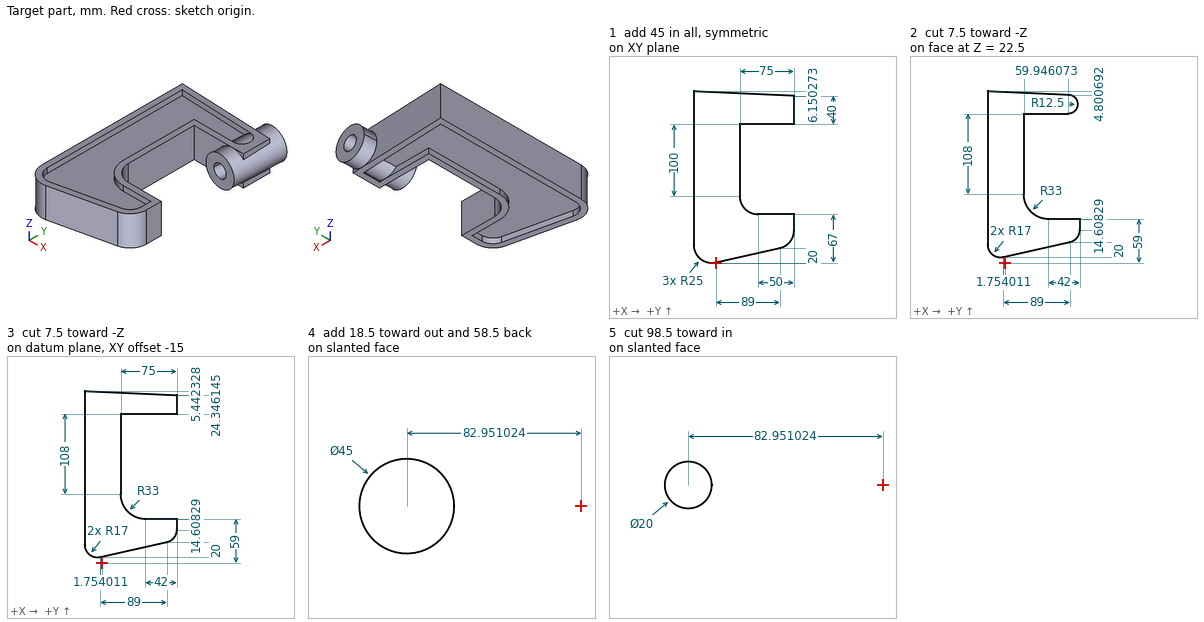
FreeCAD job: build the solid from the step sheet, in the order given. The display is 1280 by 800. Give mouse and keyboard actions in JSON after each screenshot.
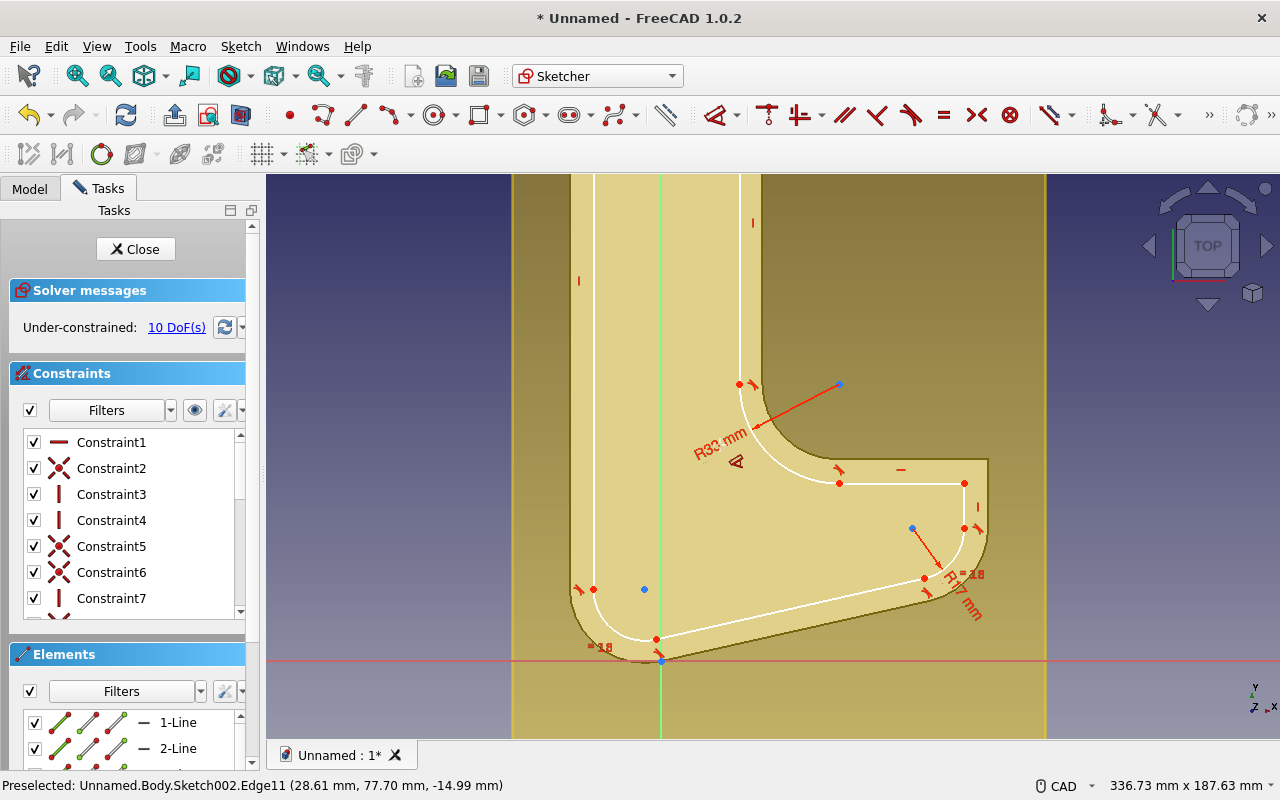
{"action": "left_click", "coordinate": [877, 484]}
{"action": "left_click", "coordinate": [902, 518]}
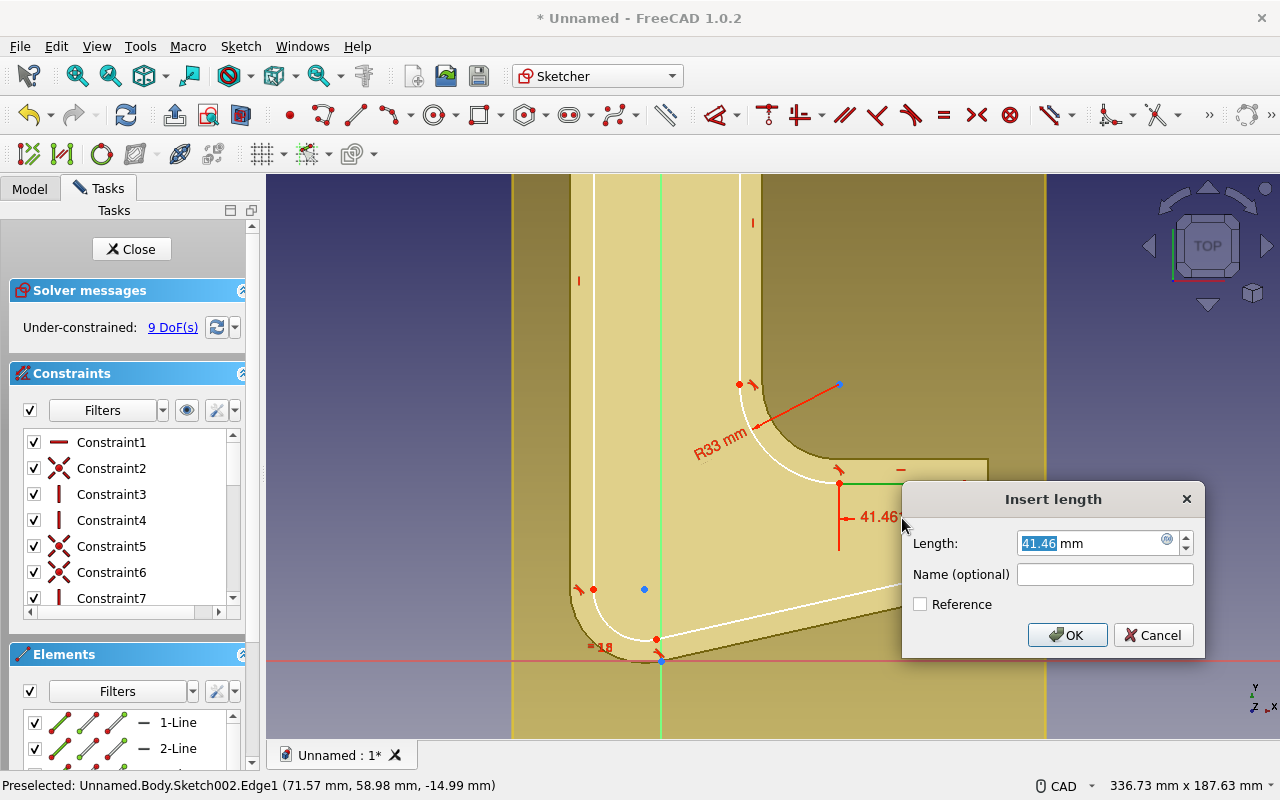
{"action": "type", "text": "42"}
{"action": "key", "text": "Return"}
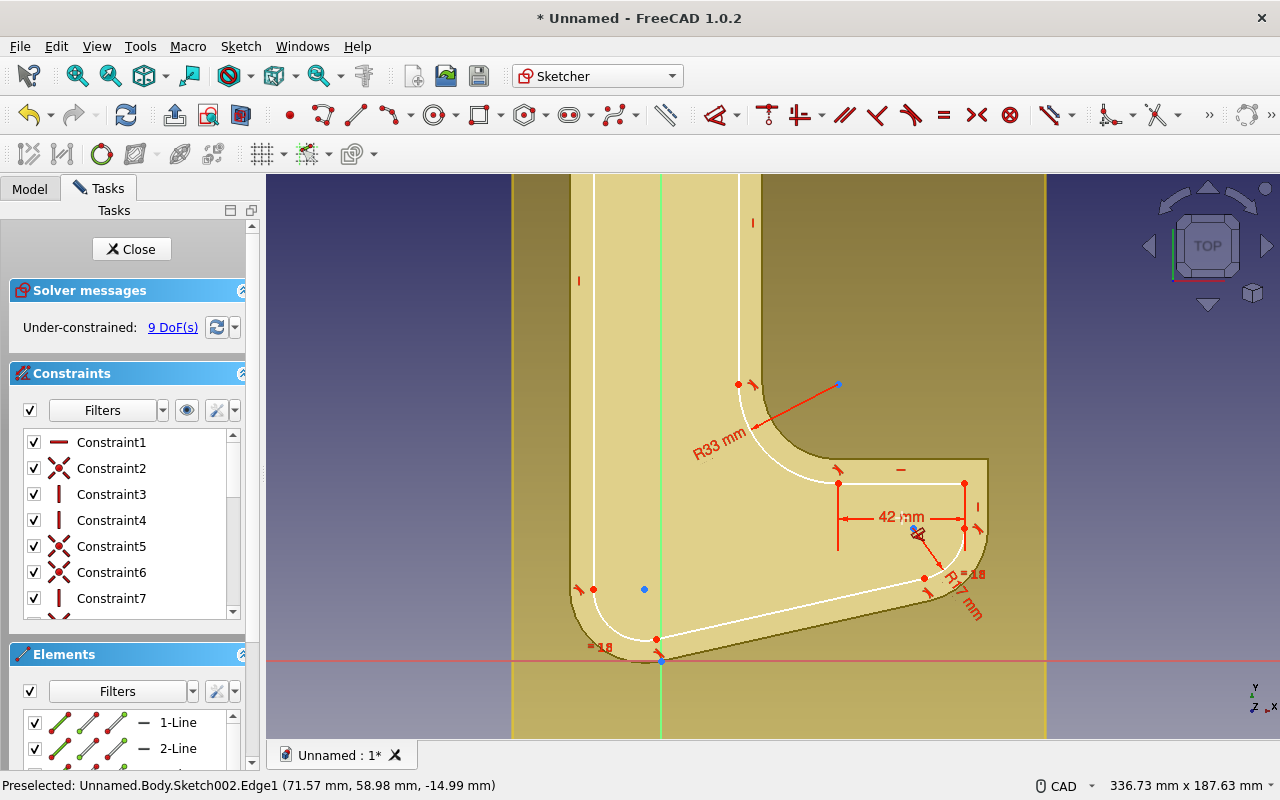
{"action": "scroll", "coordinate": [614, 628], "scroll_direction": "down", "scroll_amount": 3}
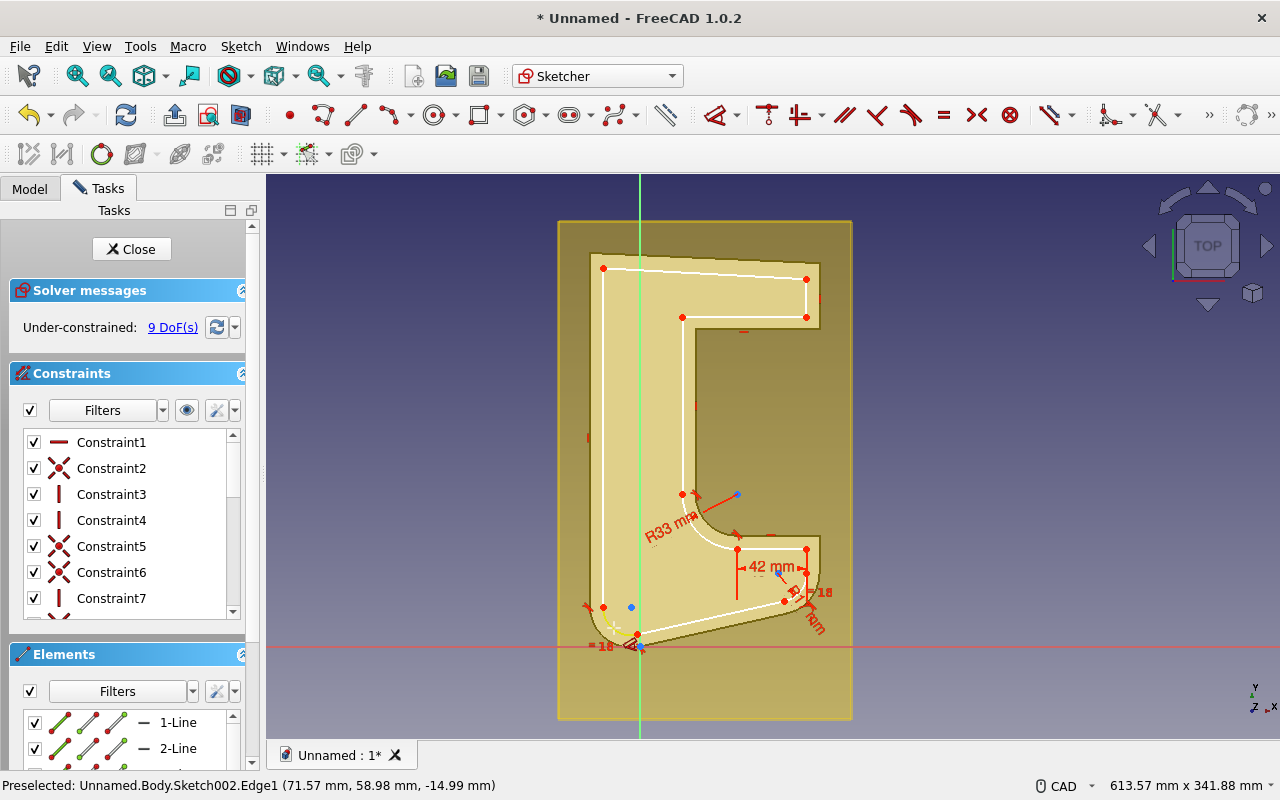
{"action": "left_click", "coordinate": [769, 317]}
{"action": "left_click", "coordinate": [744, 351]}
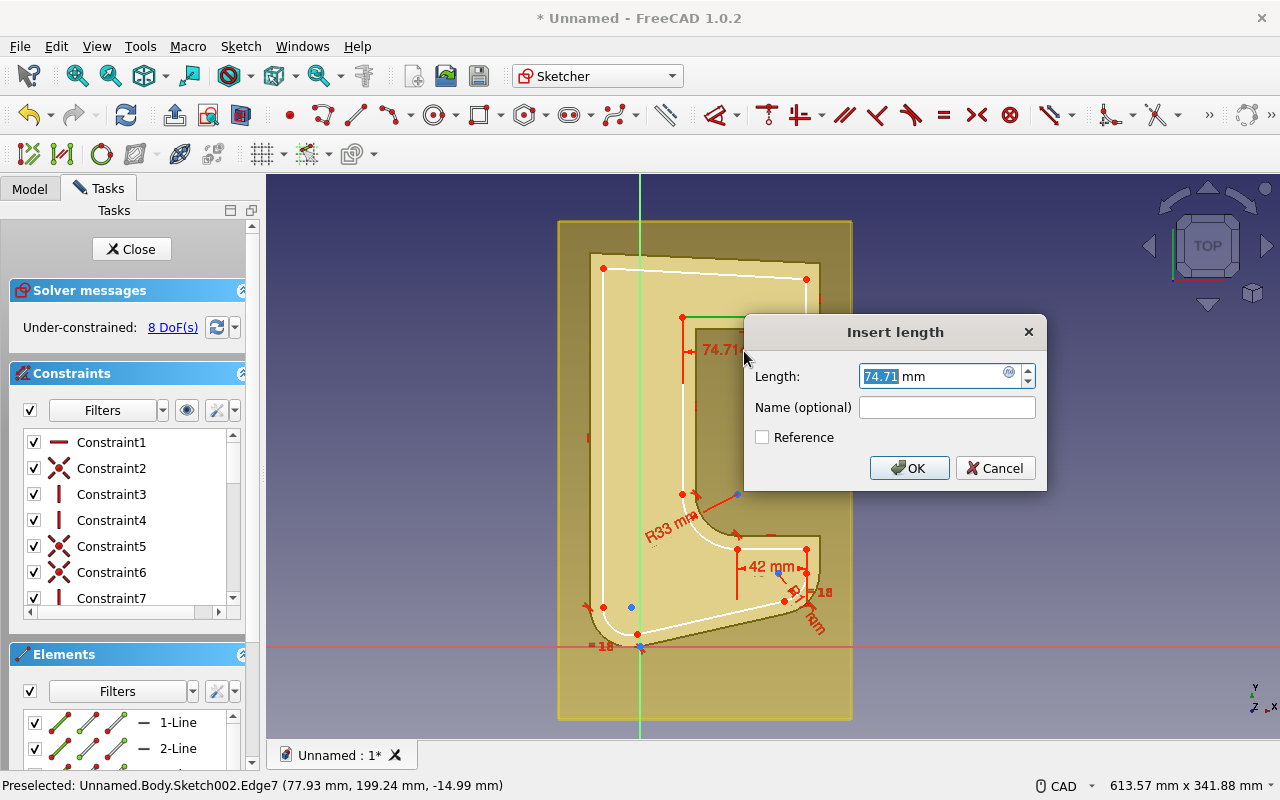
{"action": "type", "text": "75"}
{"action": "key", "text": "Return"}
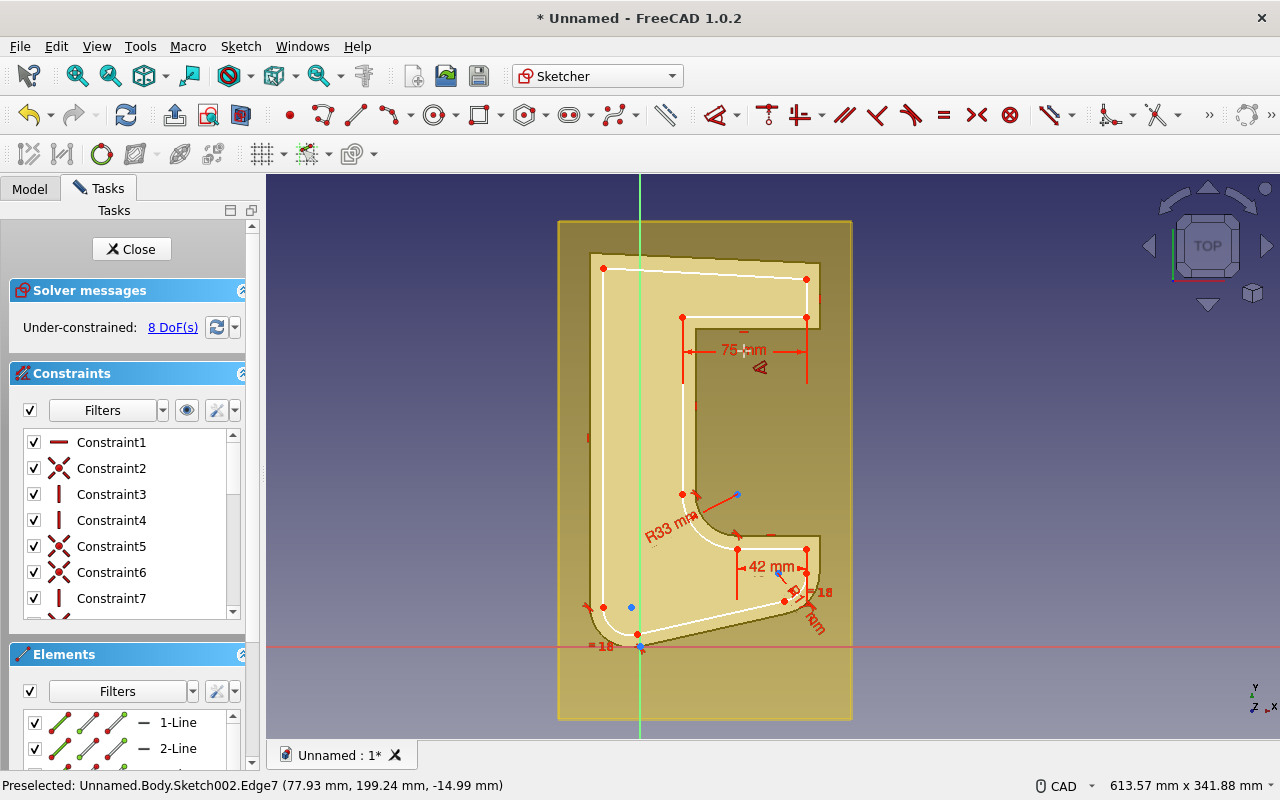
{"action": "left_click", "coordinate": [683, 370]}
{"action": "left_click", "coordinate": [717, 406]}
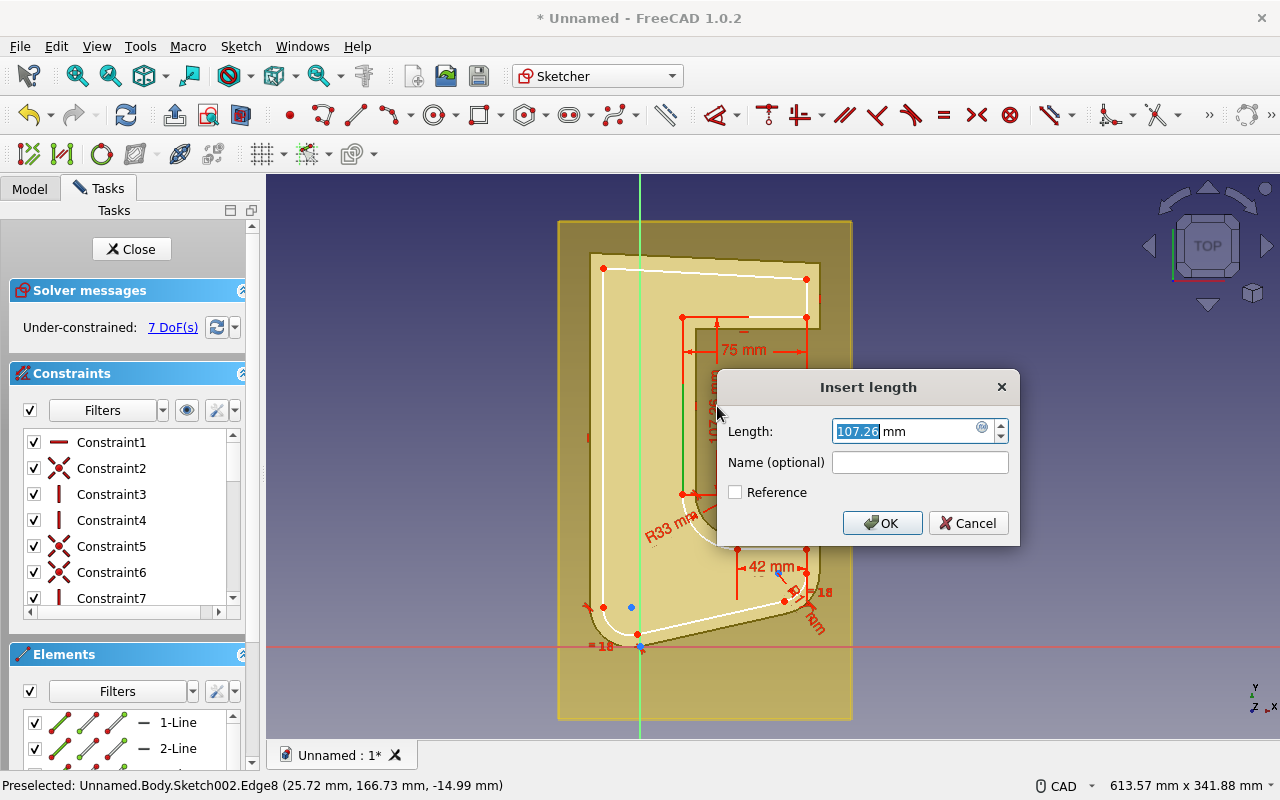
{"action": "type", "text": "108"}
{"action": "key", "text": "Return"}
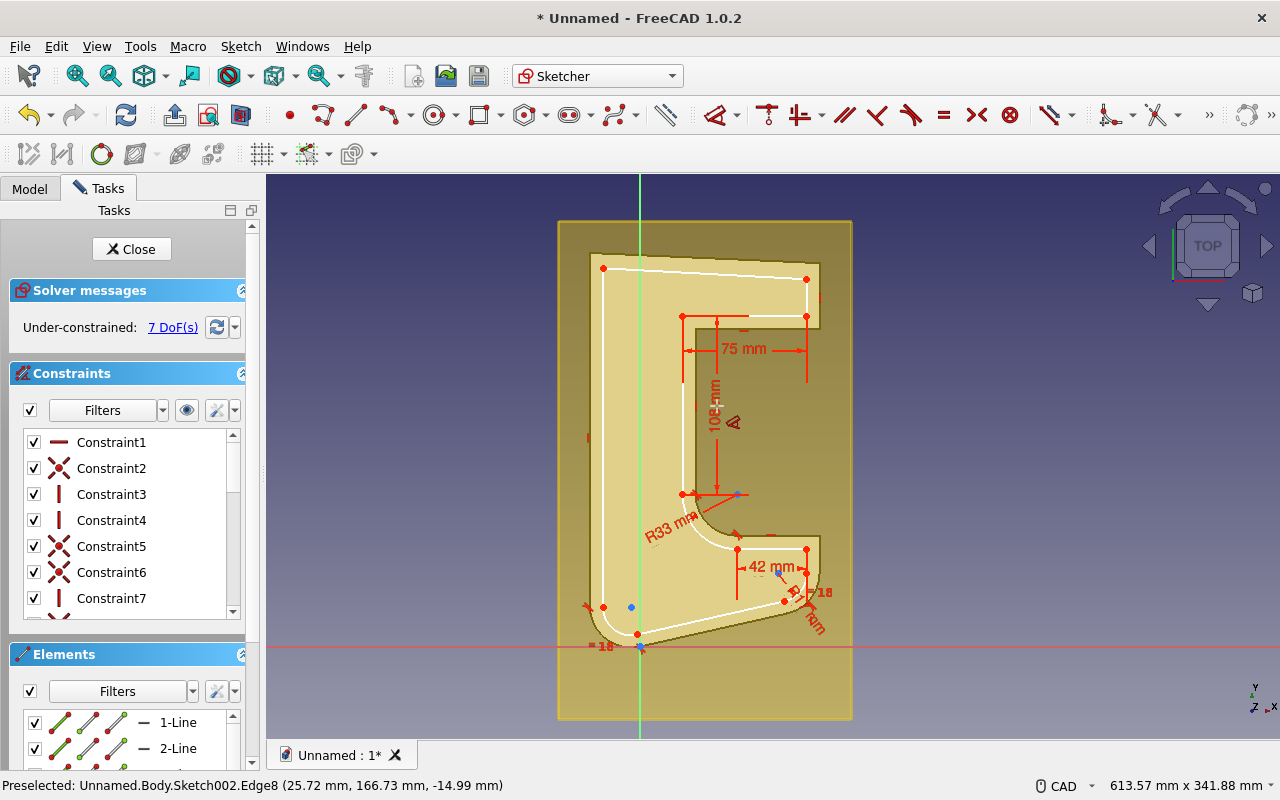
{"action": "left_click", "coordinate": [737, 549]}
{"action": "left_click", "coordinate": [771, 632]}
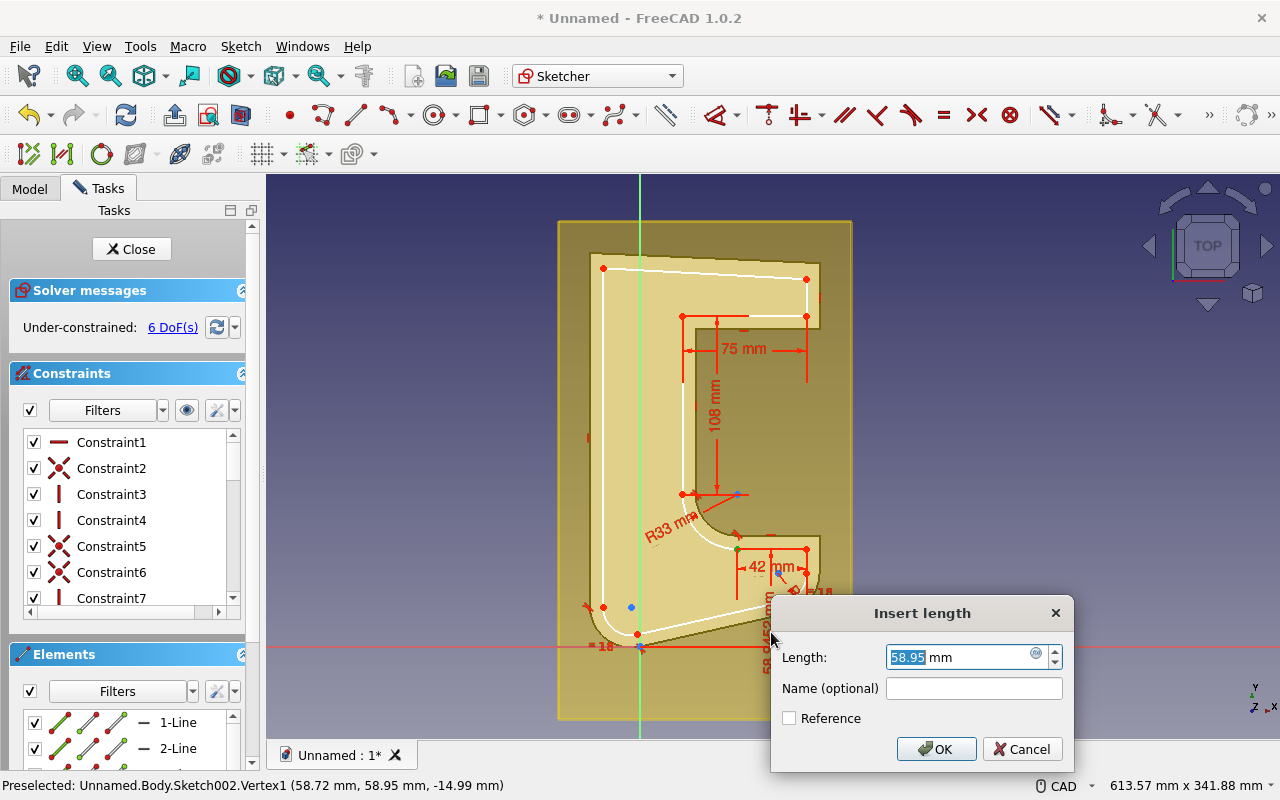
{"action": "type", "text": "59"}
{"action": "key", "text": "Return"}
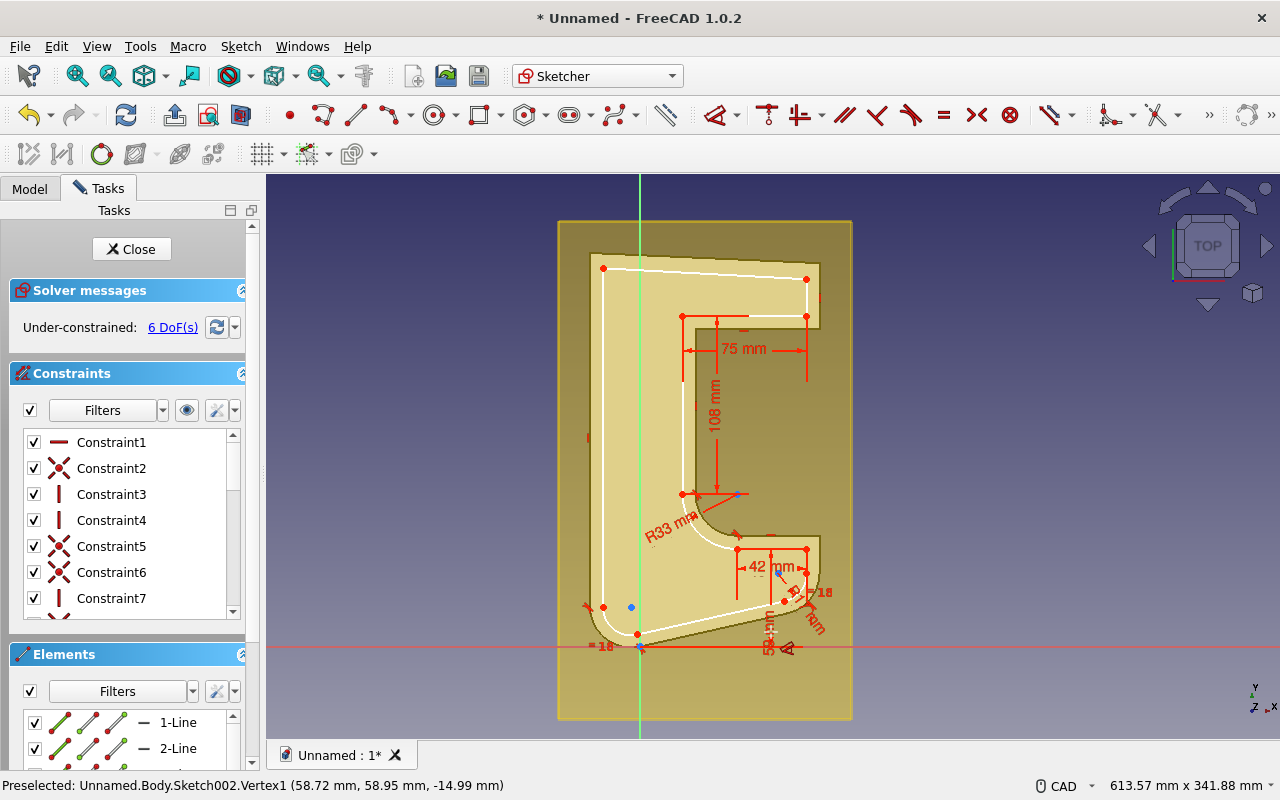
{"action": "left_click", "coordinate": [741, 611]}
{"action": "left_click", "coordinate": [711, 669]}